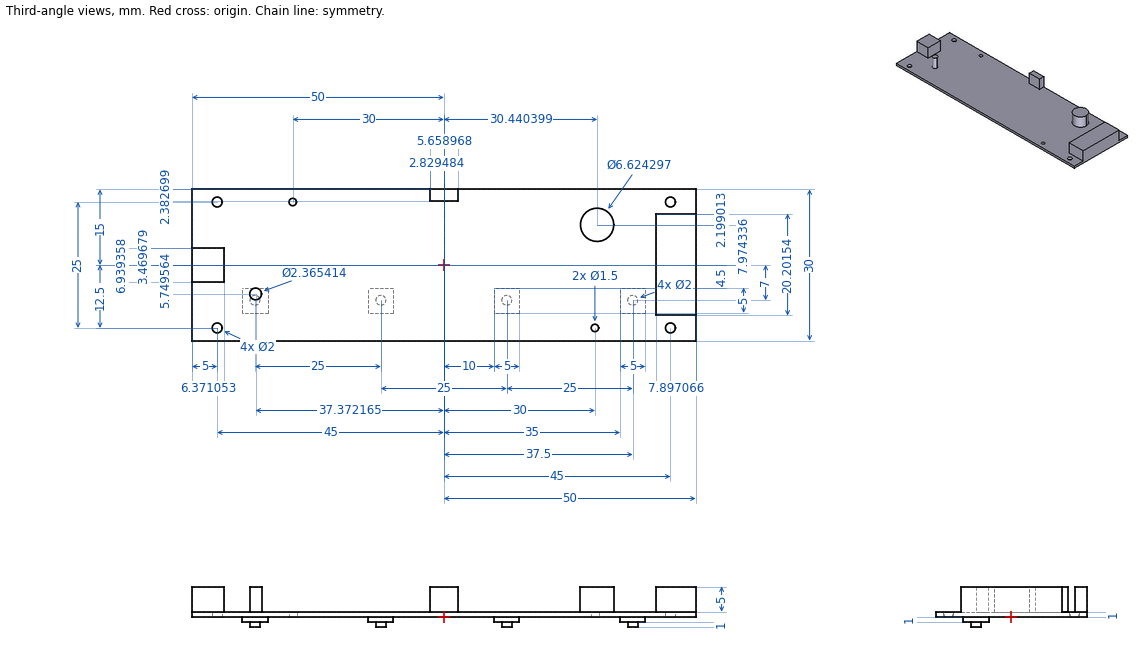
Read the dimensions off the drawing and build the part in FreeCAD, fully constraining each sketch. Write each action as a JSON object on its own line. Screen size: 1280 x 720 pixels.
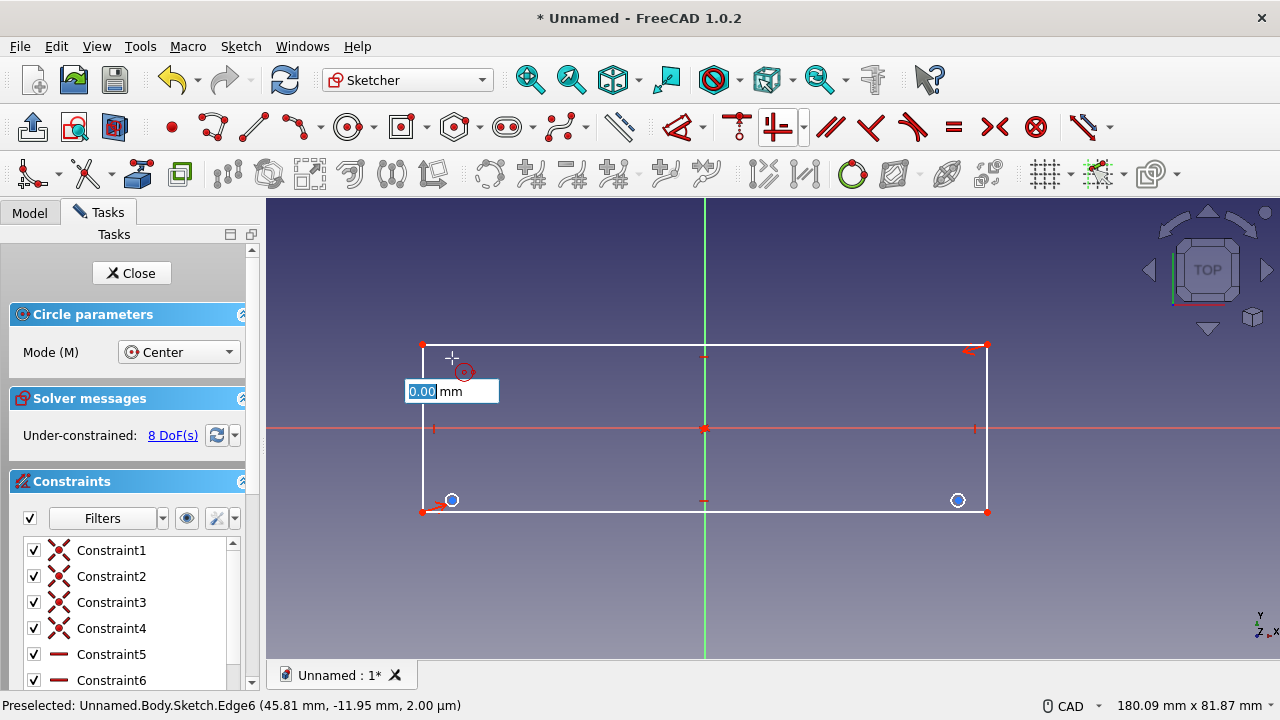
{"action": "scroll", "coordinate": [455, 362], "scroll_direction": "up", "scroll_amount": 6}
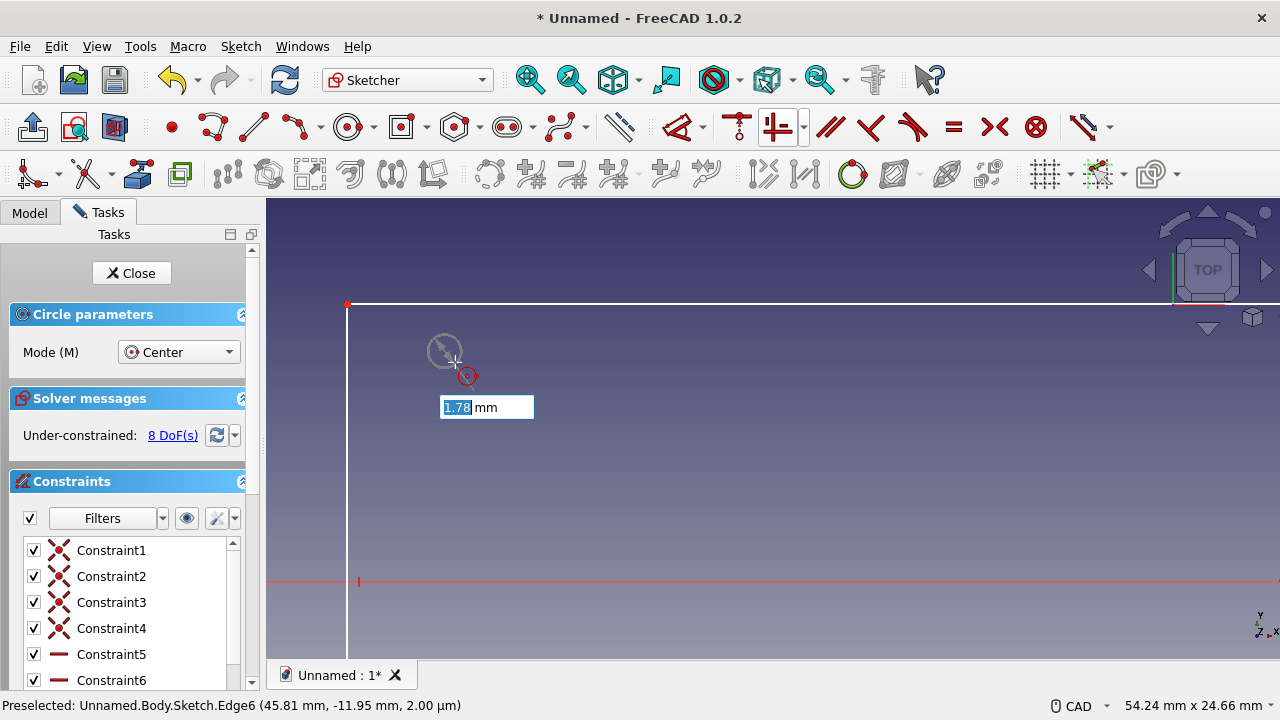
{"action": "left_click", "coordinate": [456, 361]}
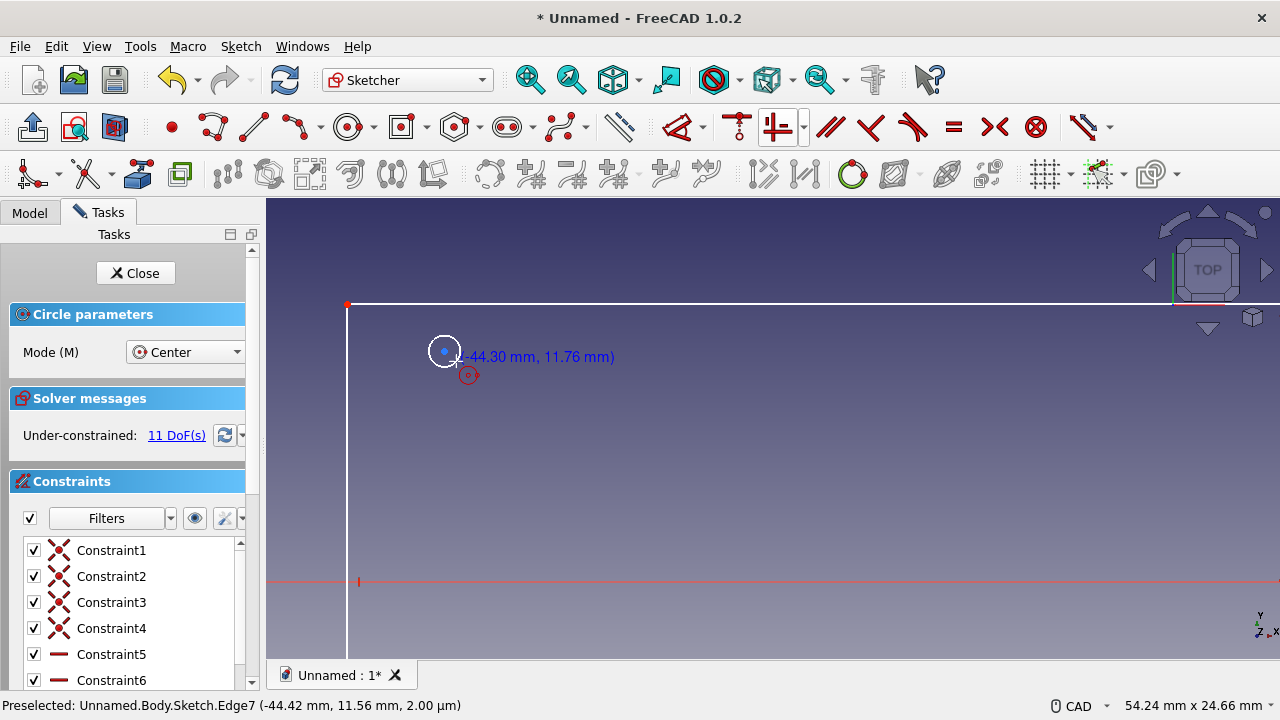
{"action": "scroll", "coordinate": [455, 362], "scroll_direction": "down", "scroll_amount": 6}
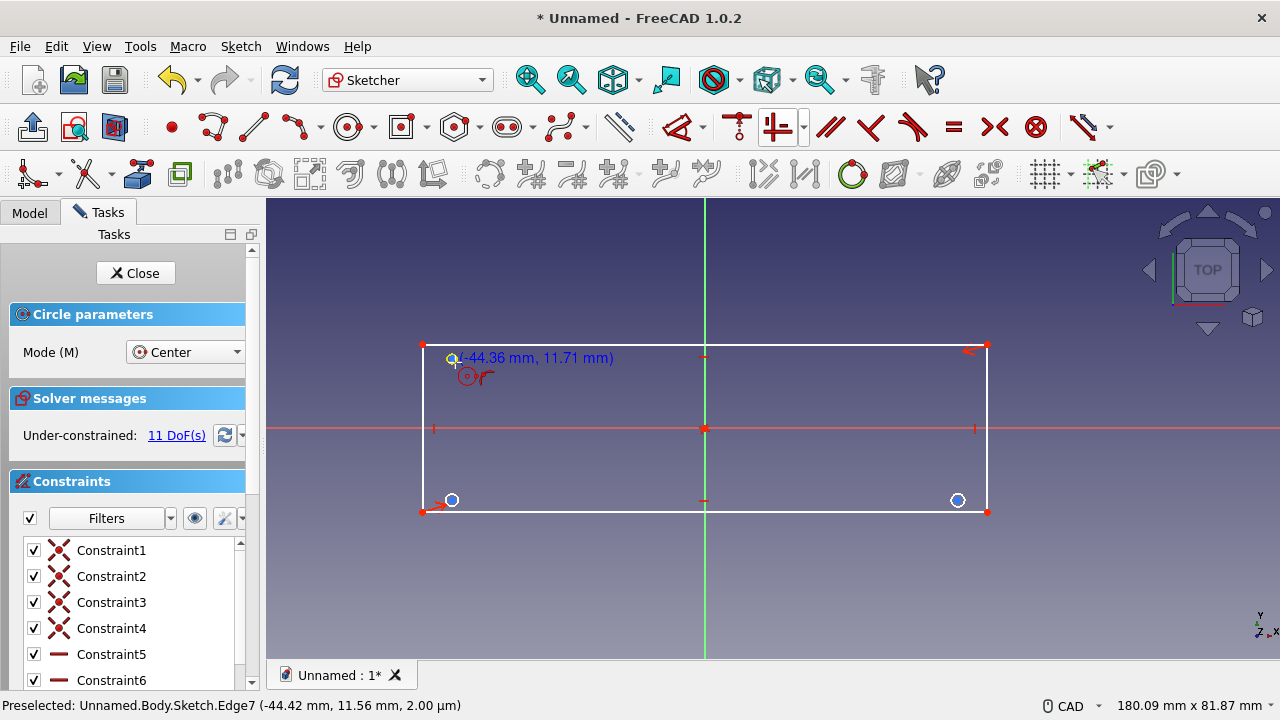
{"action": "scroll", "coordinate": [958, 358], "scroll_direction": "up", "scroll_amount": 7}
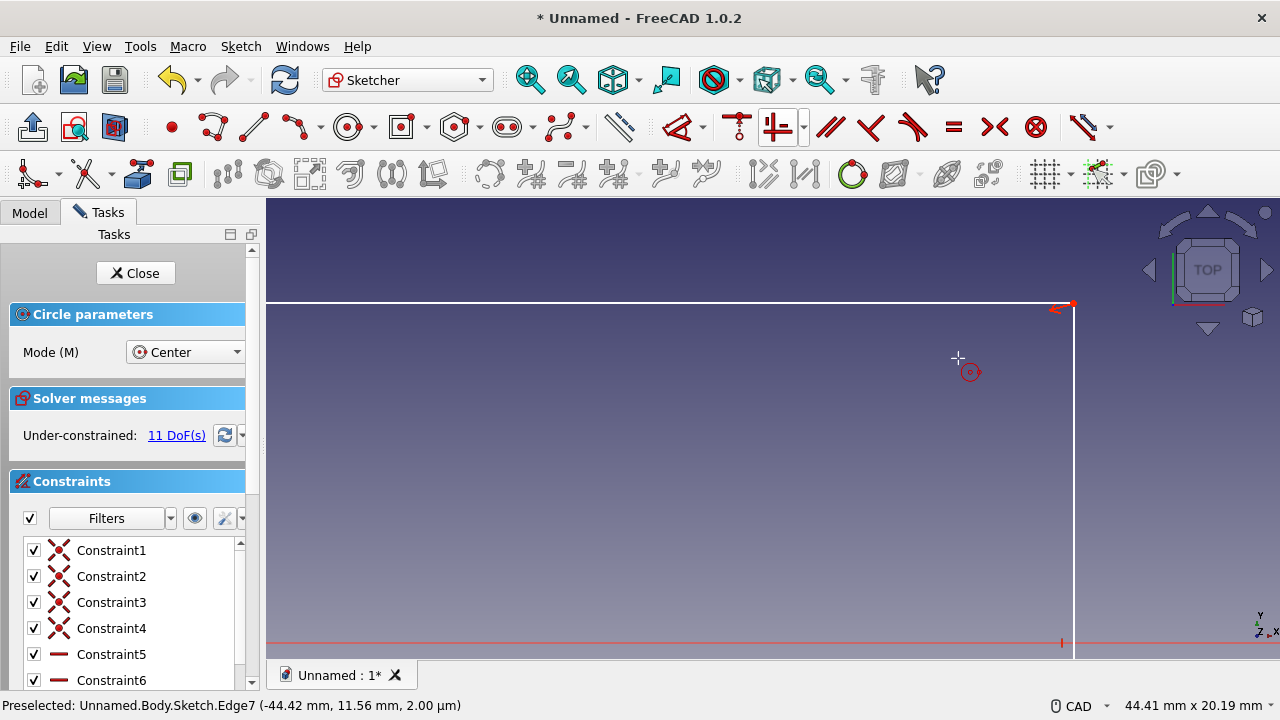
{"action": "scroll", "coordinate": [958, 358], "scroll_direction": "down", "scroll_amount": 7}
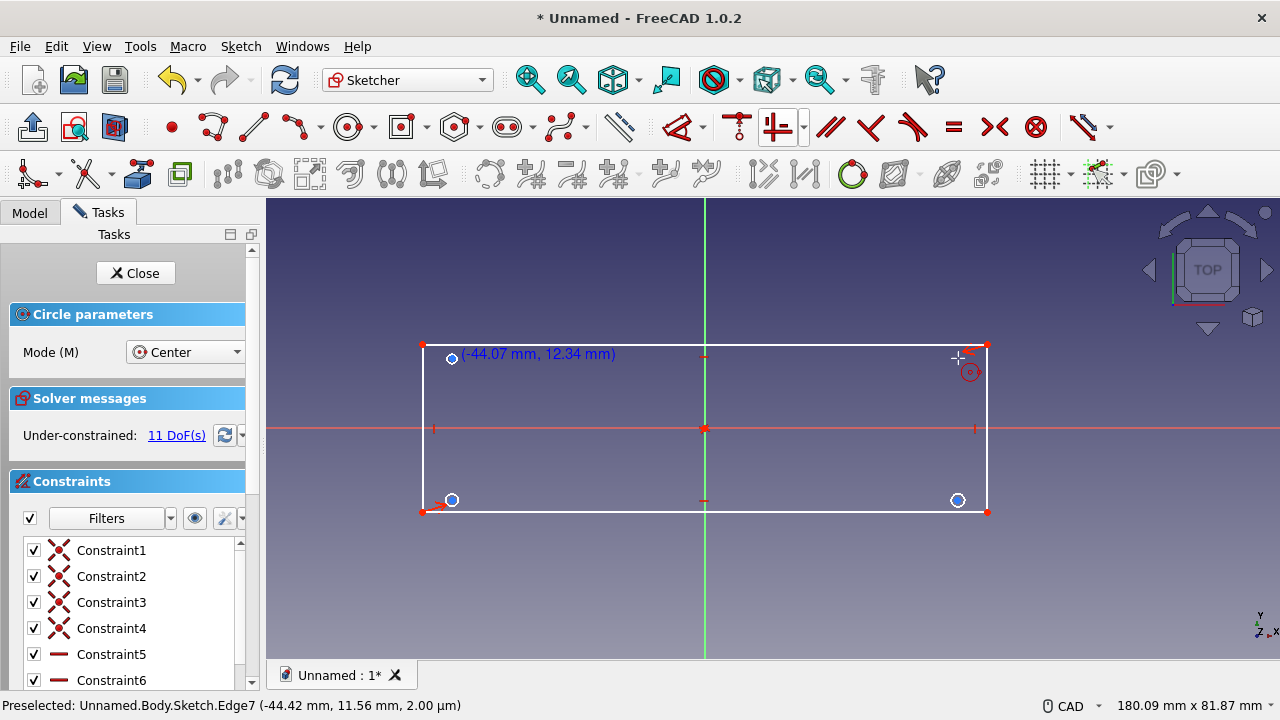
{"action": "left_click", "coordinate": [958, 358]}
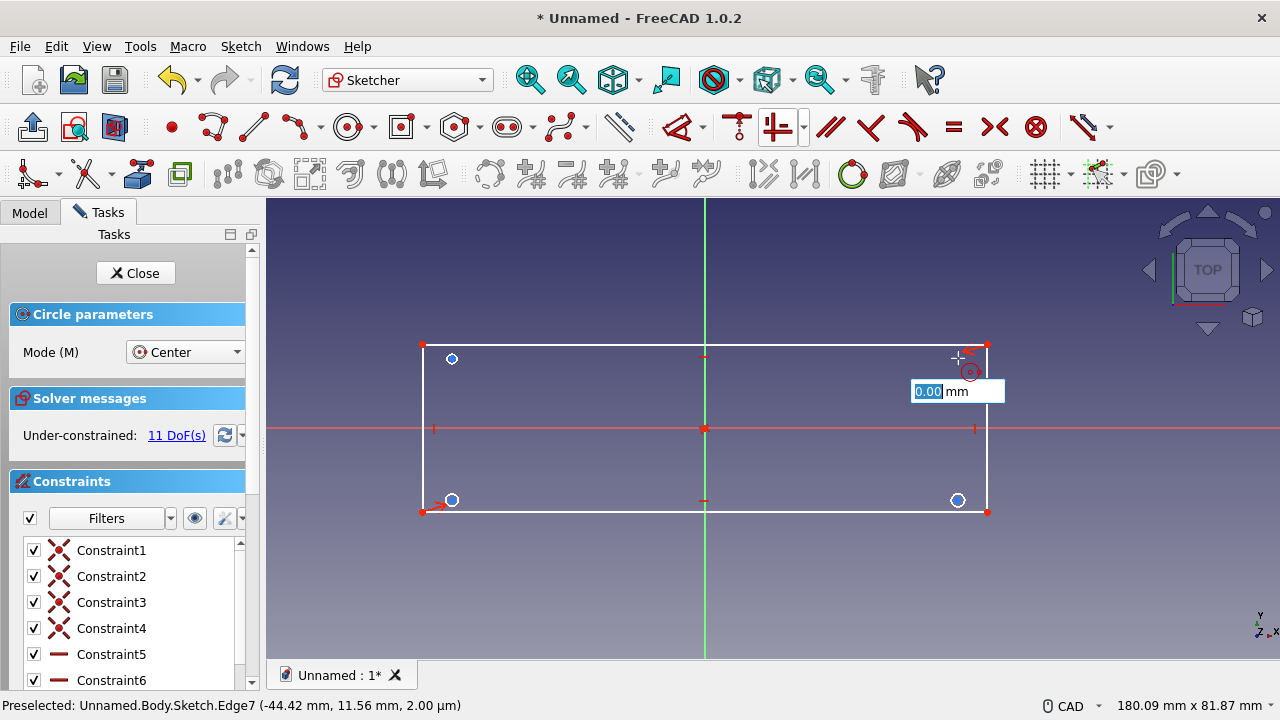
{"action": "scroll", "coordinate": [962, 362], "scroll_direction": "up", "scroll_amount": 6}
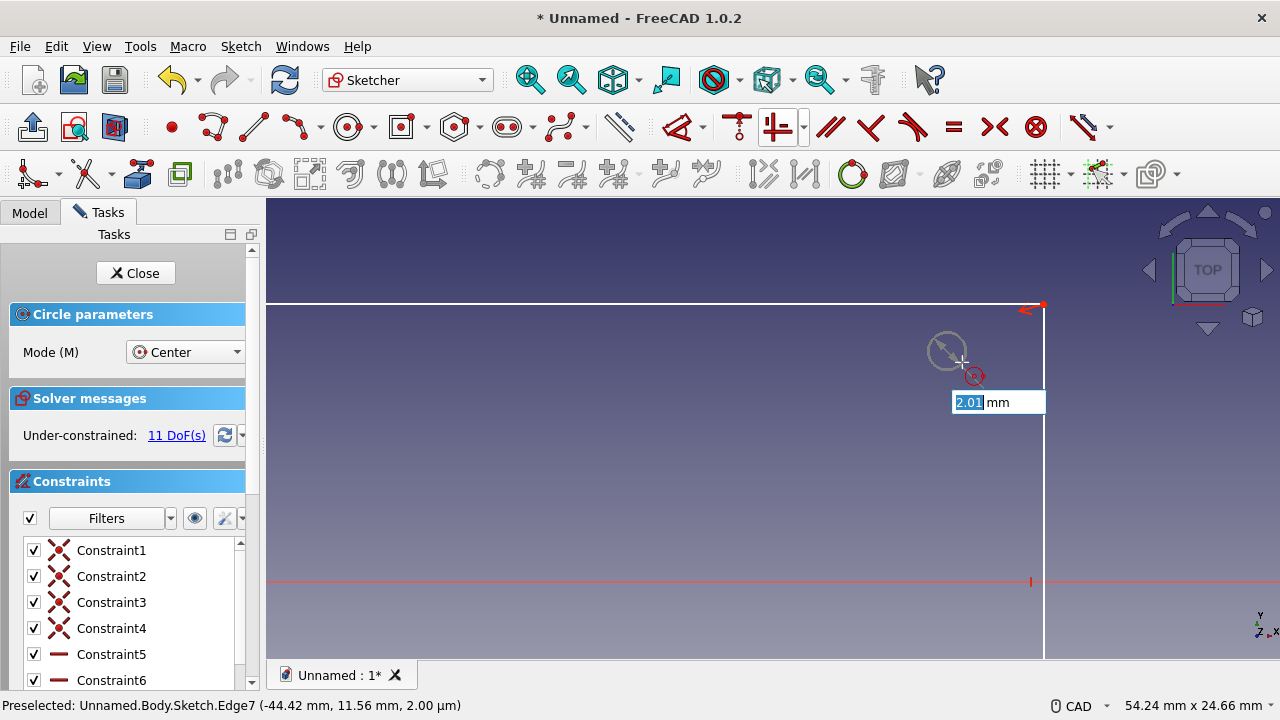
{"action": "left_click", "coordinate": [961, 361]}
{"action": "key", "text": "Escape"}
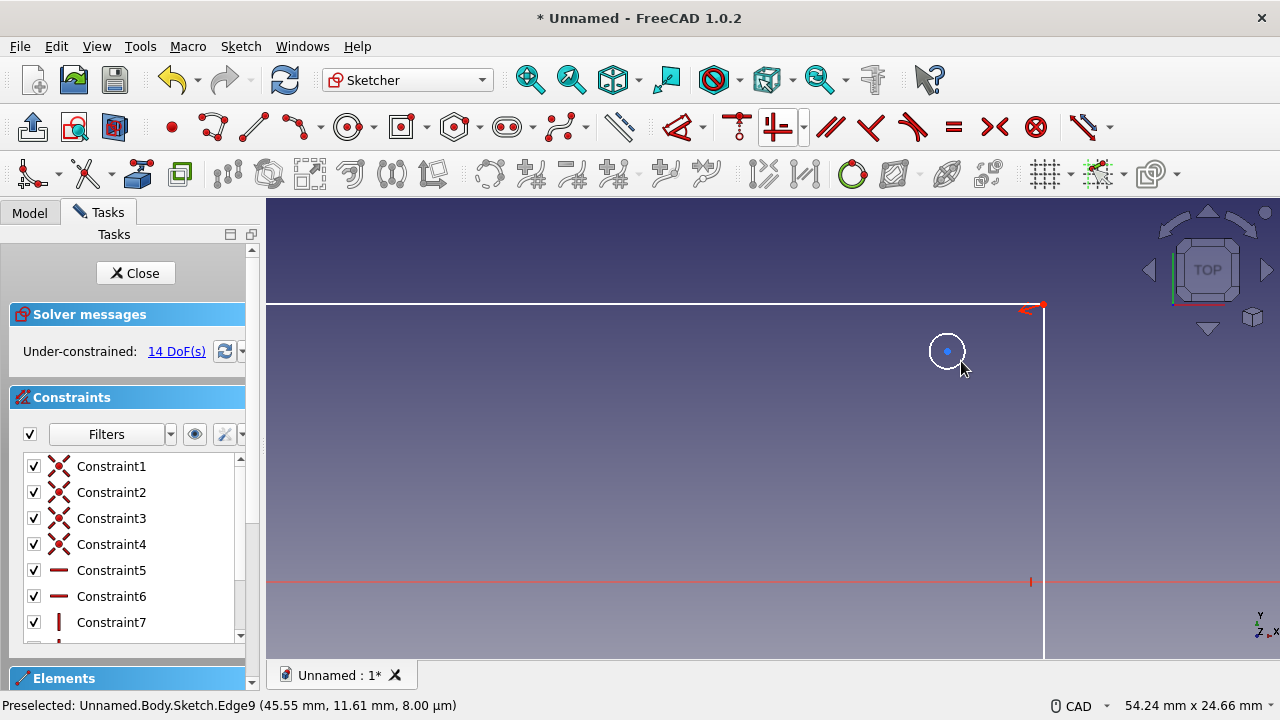
{"action": "scroll", "coordinate": [962, 362], "scroll_direction": "down", "scroll_amount": 6}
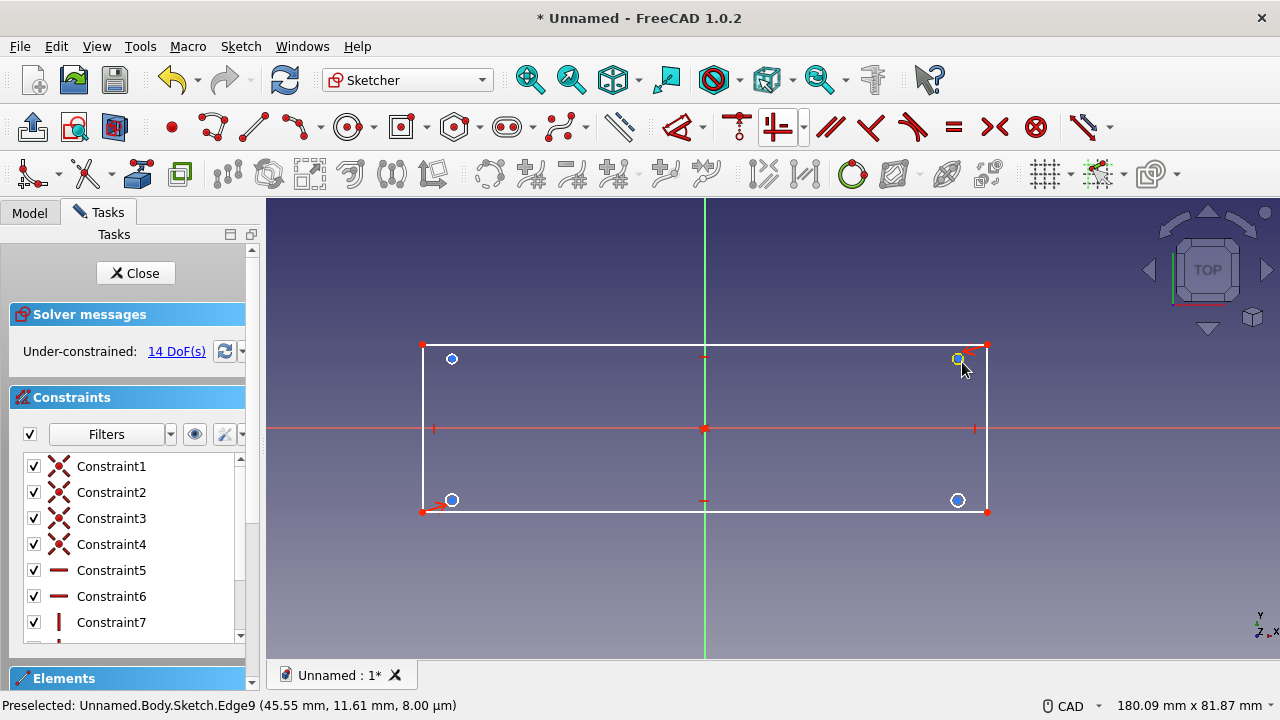
{"action": "scroll", "coordinate": [456, 496], "scroll_direction": "up", "scroll_amount": 5}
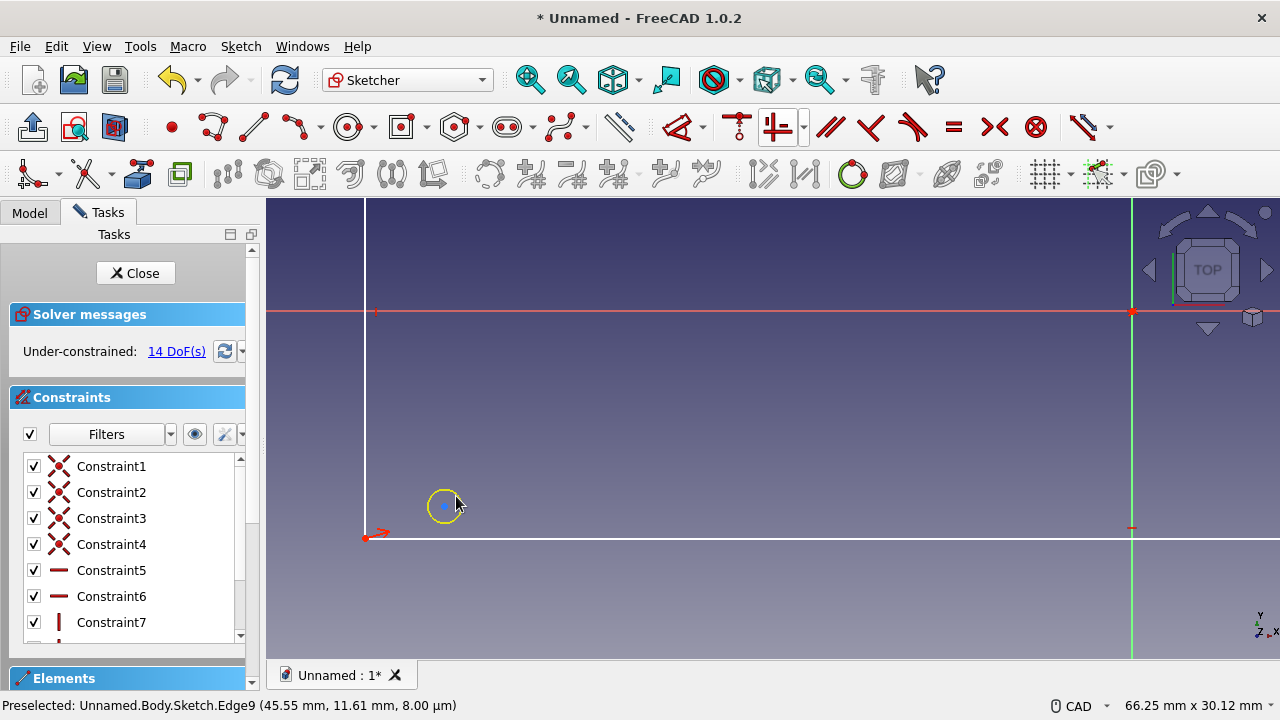
{"action": "left_click", "coordinate": [457, 494]}